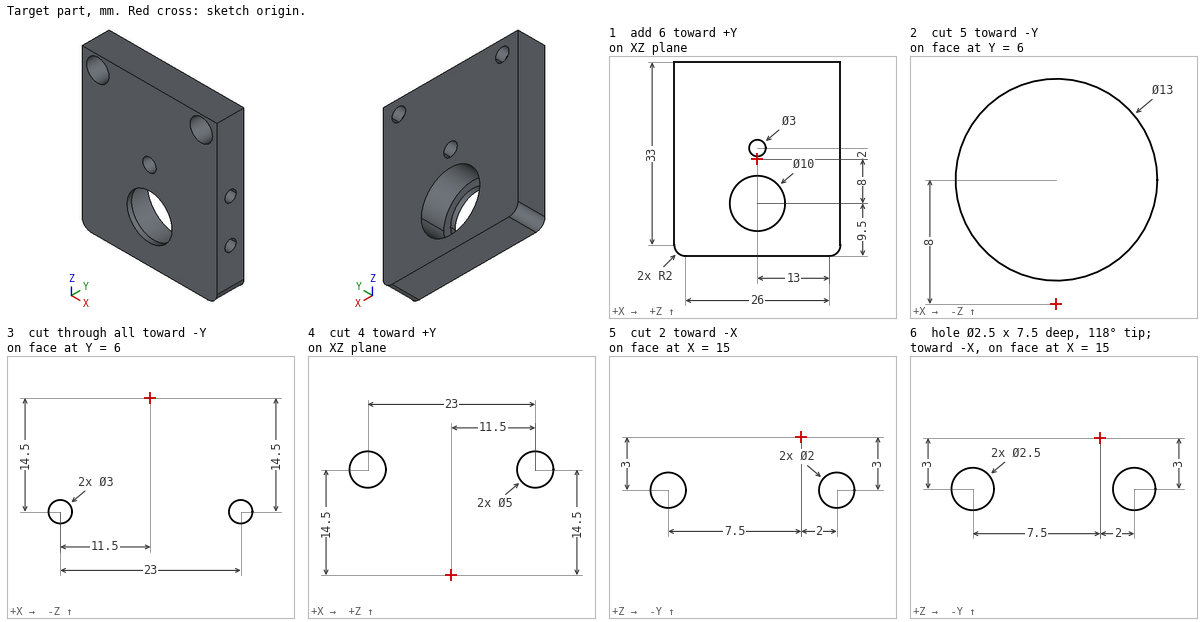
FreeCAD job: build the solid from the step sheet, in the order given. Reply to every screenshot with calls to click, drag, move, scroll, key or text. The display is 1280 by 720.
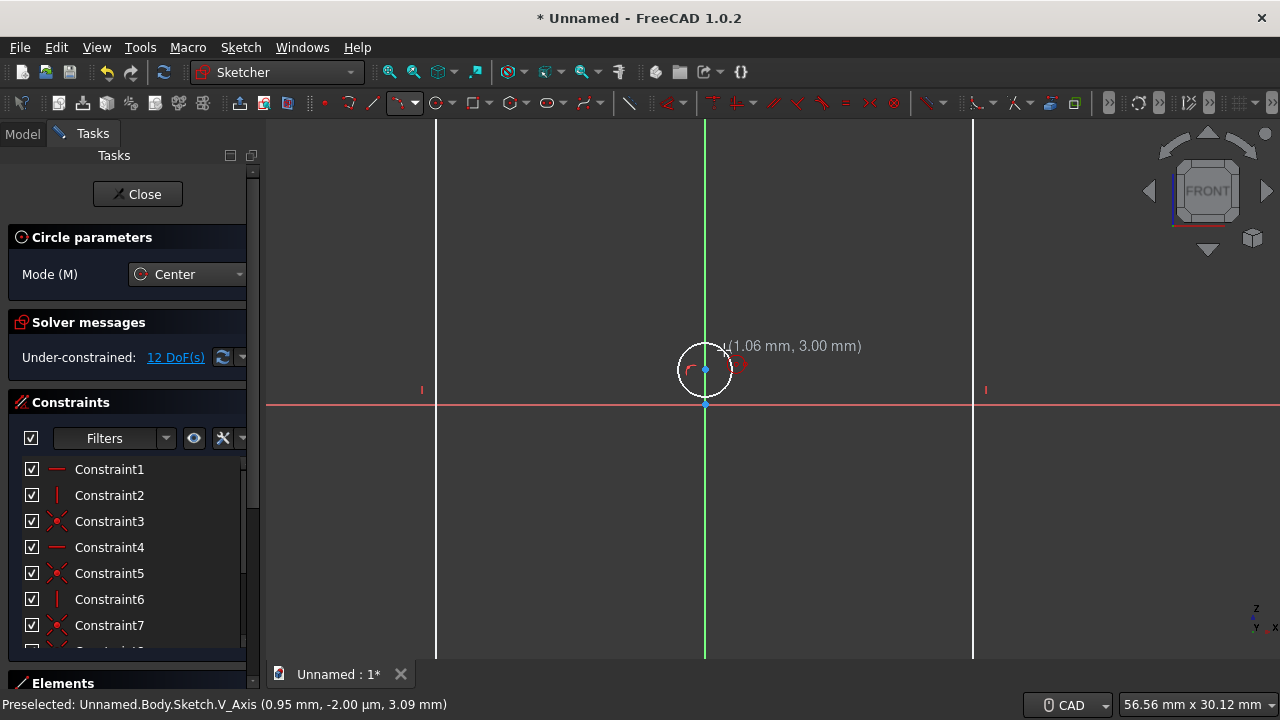
click(705, 548)
click(768, 485)
key(Escape)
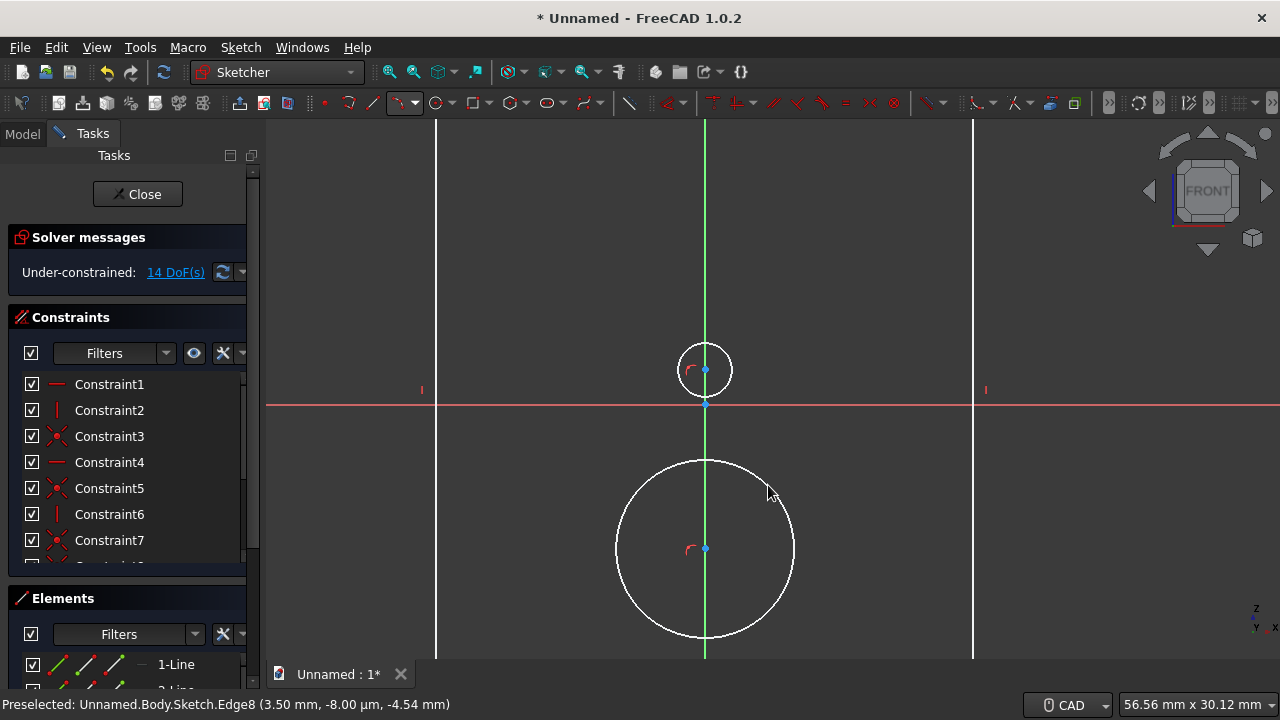
scroll(704, 370, down, 3)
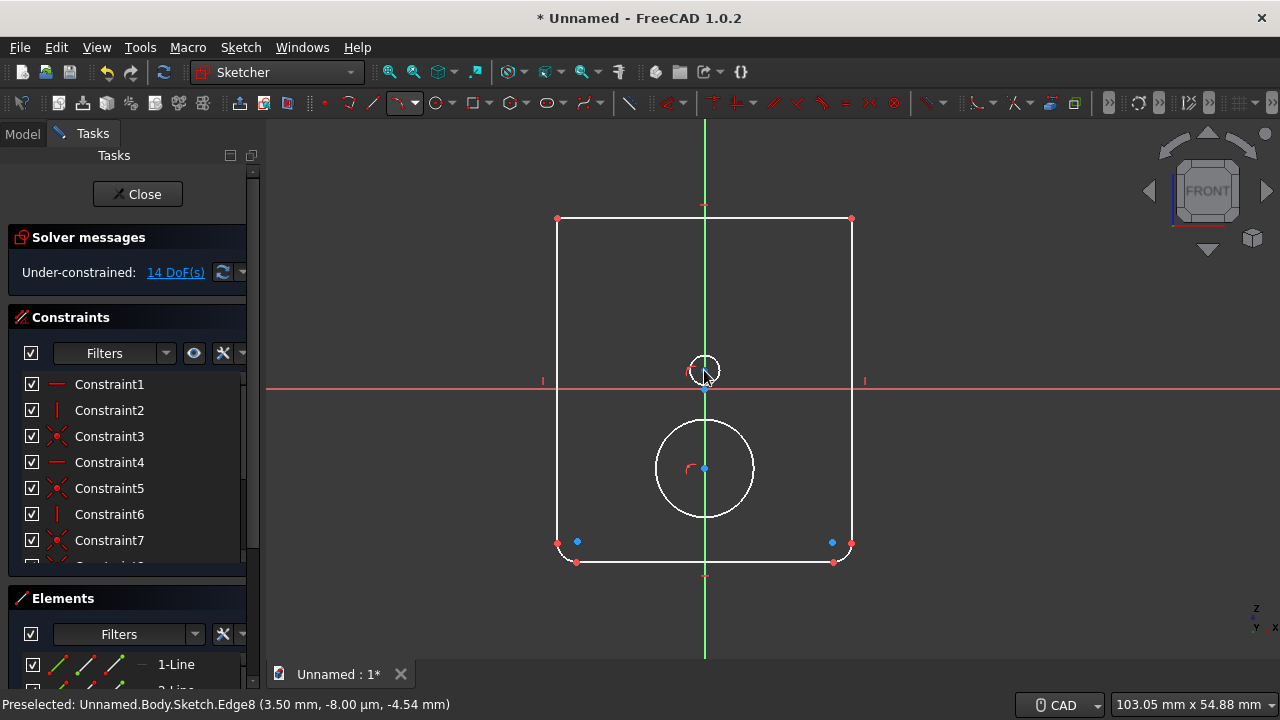
click(756, 562)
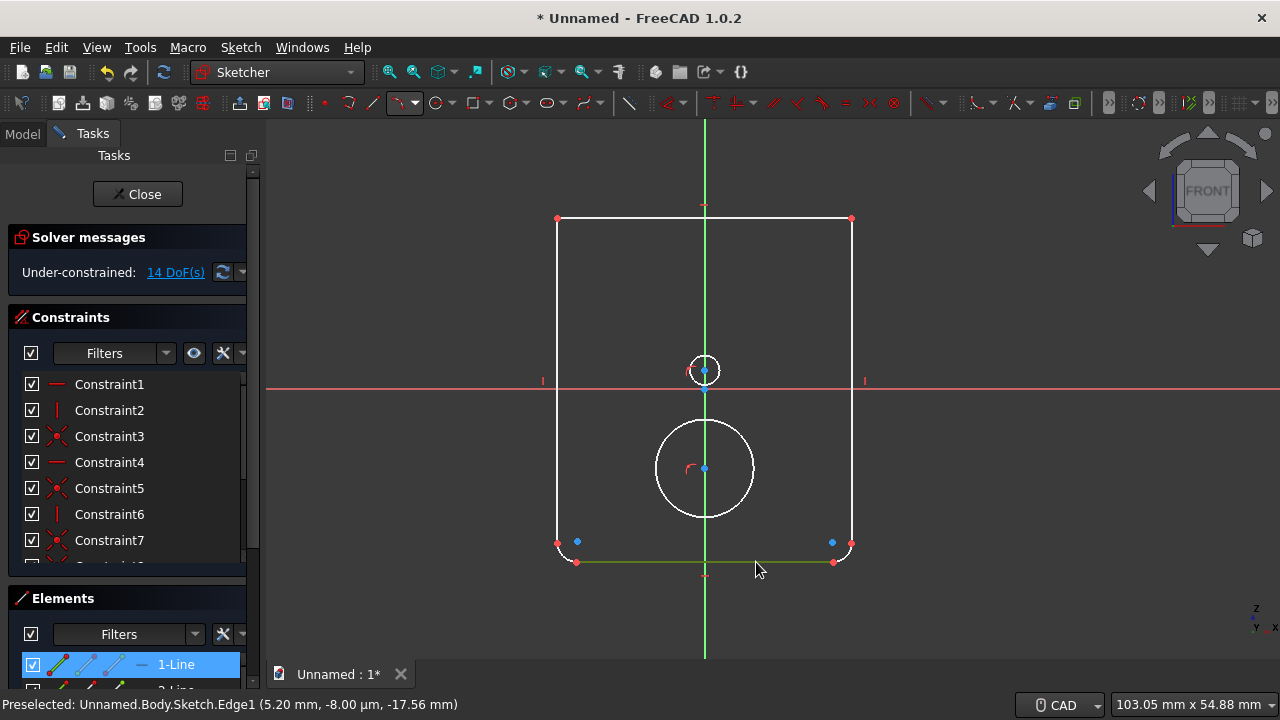
click(563, 556)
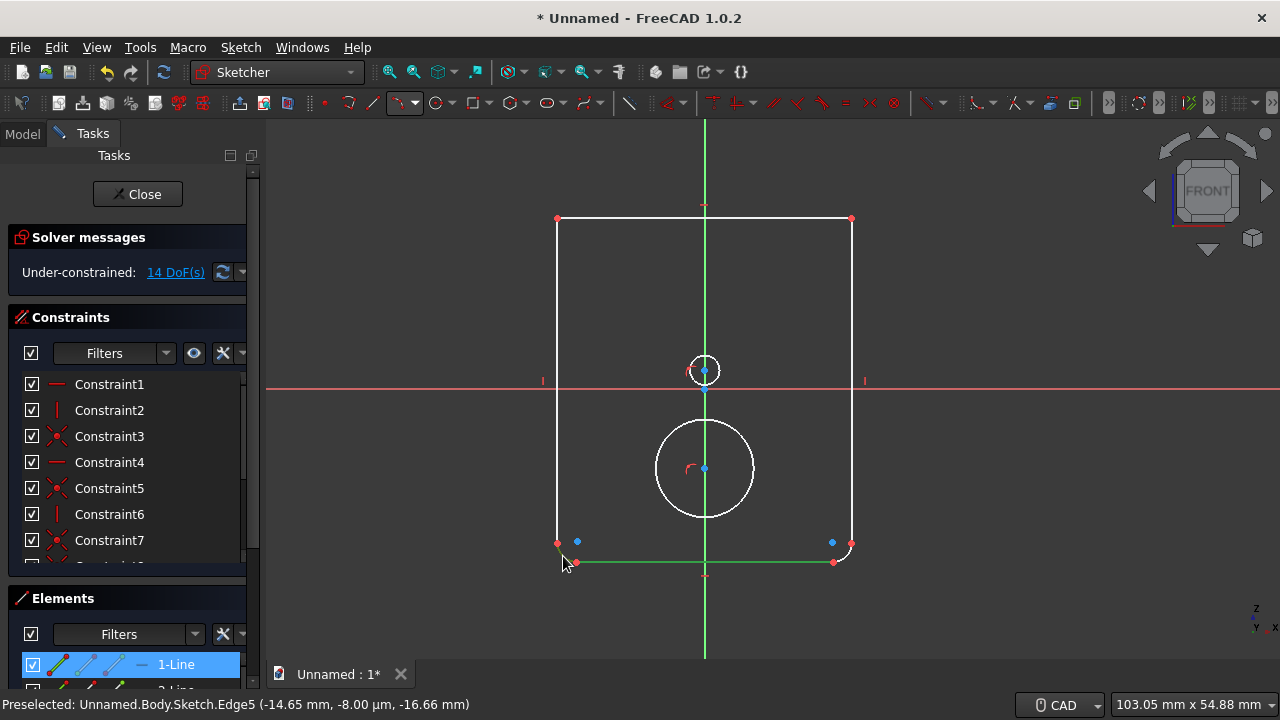
key(t)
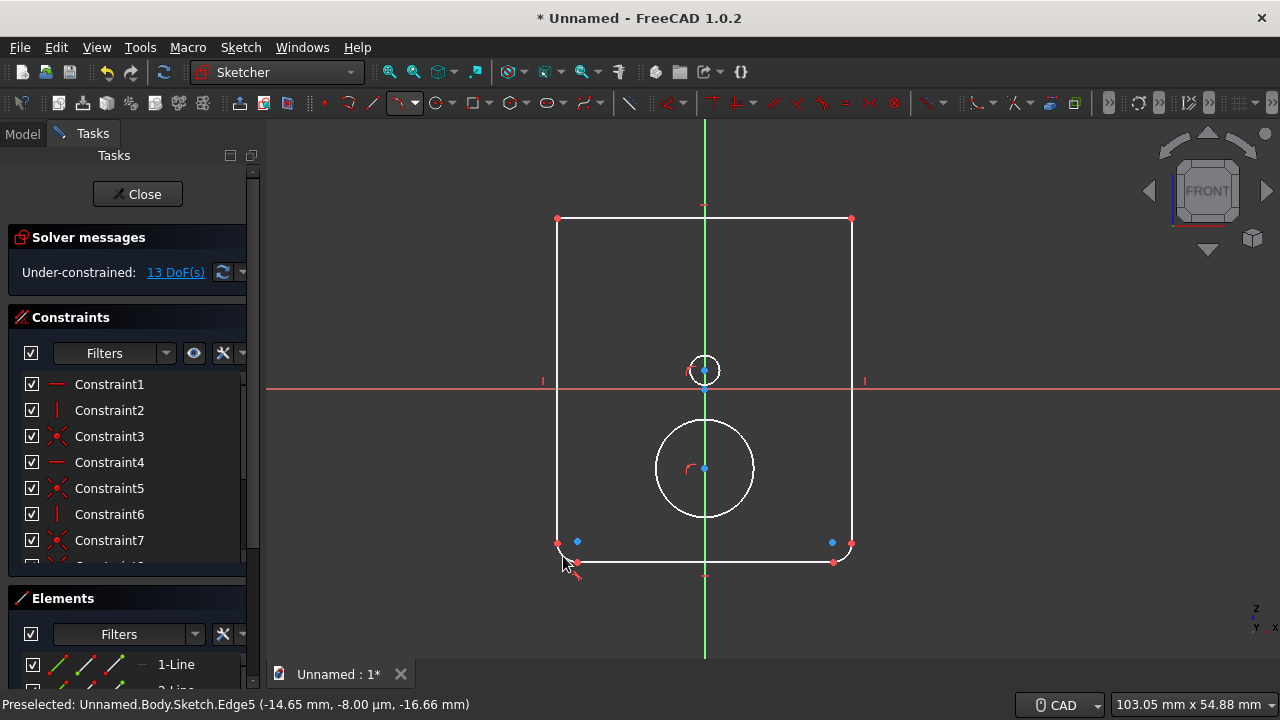
click(756, 562)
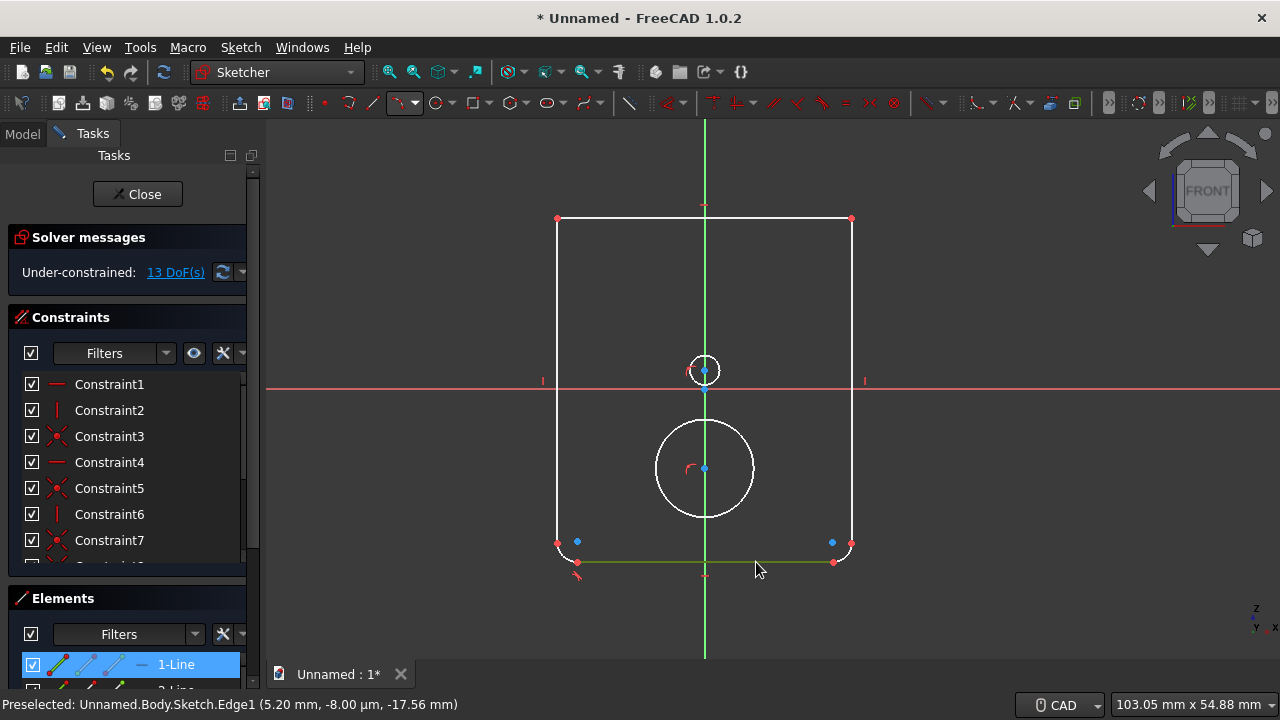
click(846, 556)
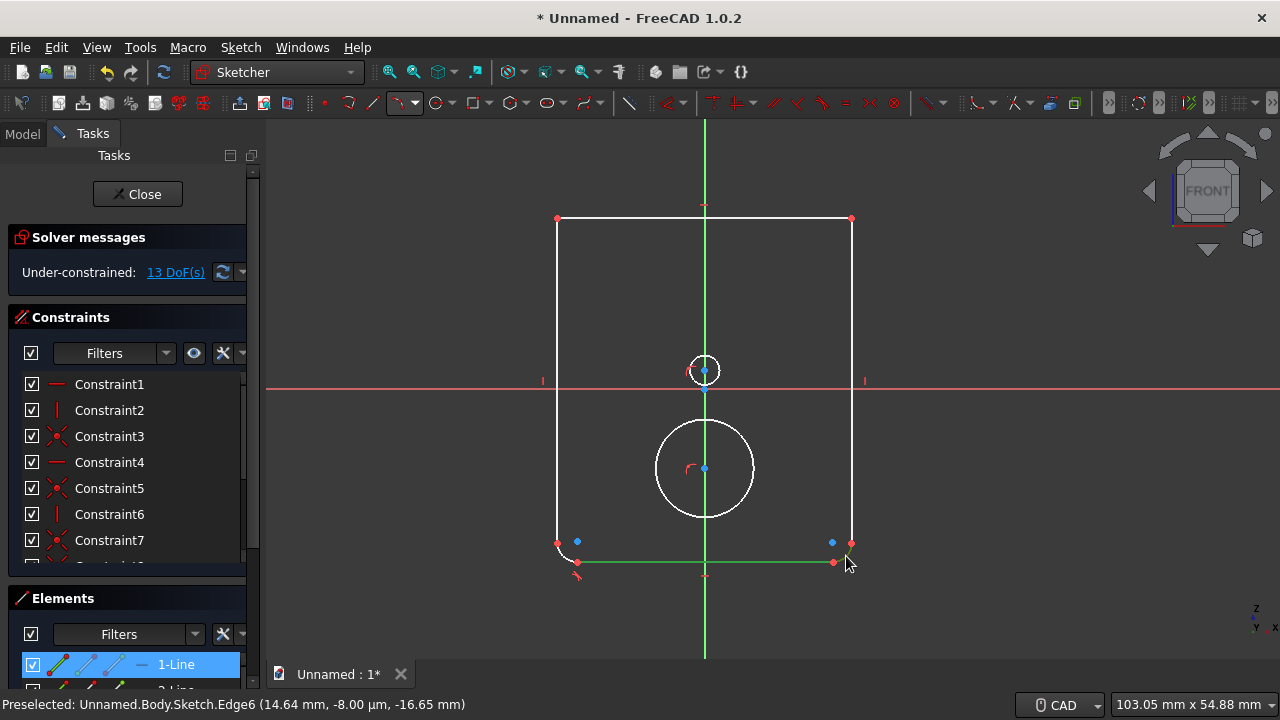
key(t)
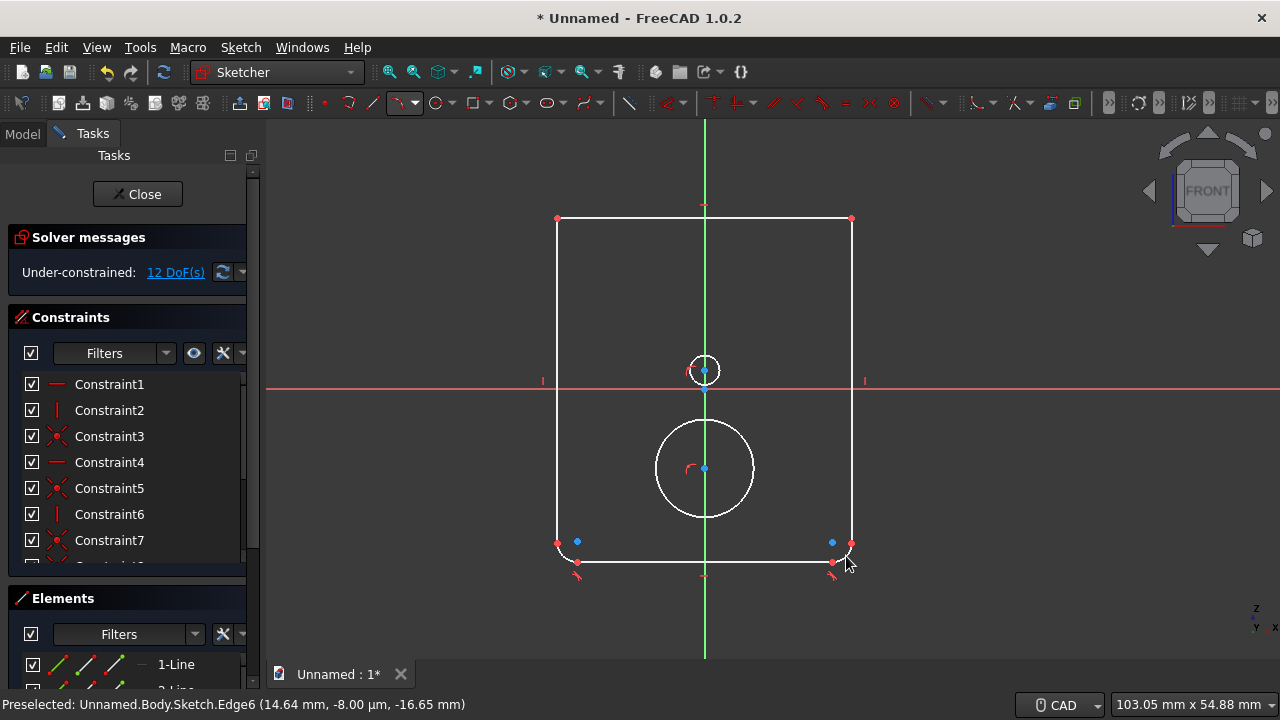
click(557, 446)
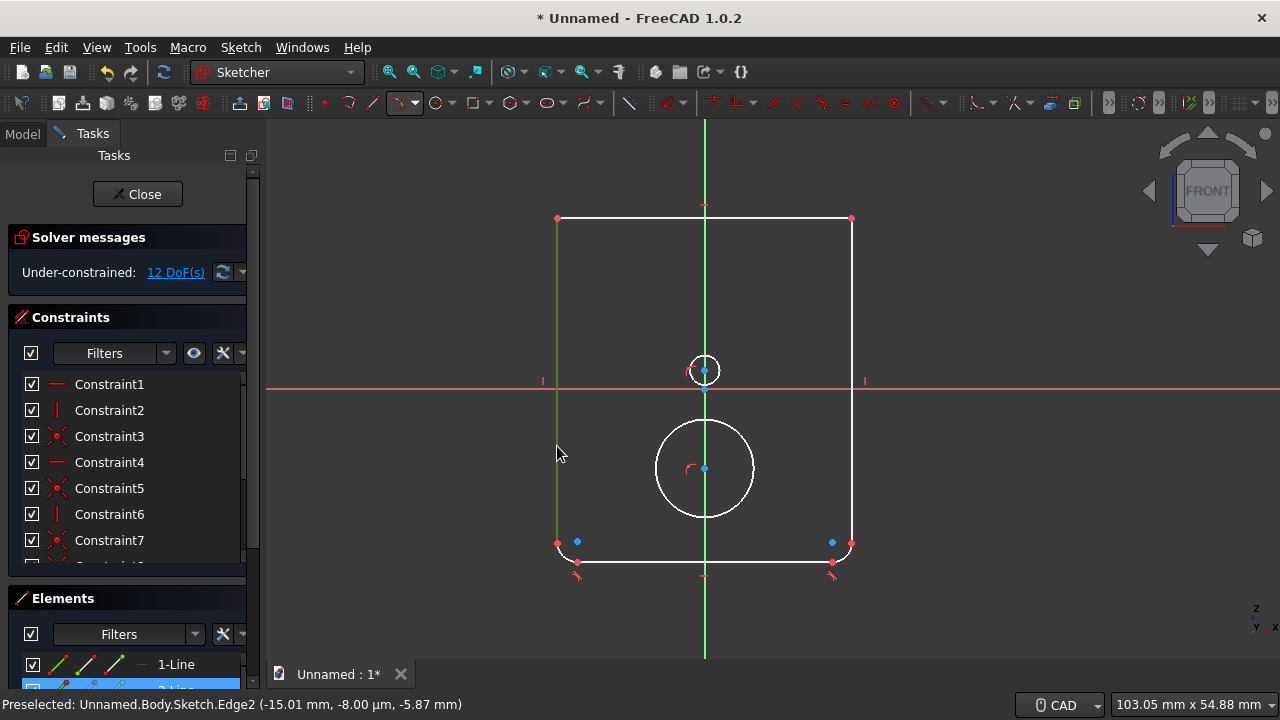
scroll(560, 552, up, 3)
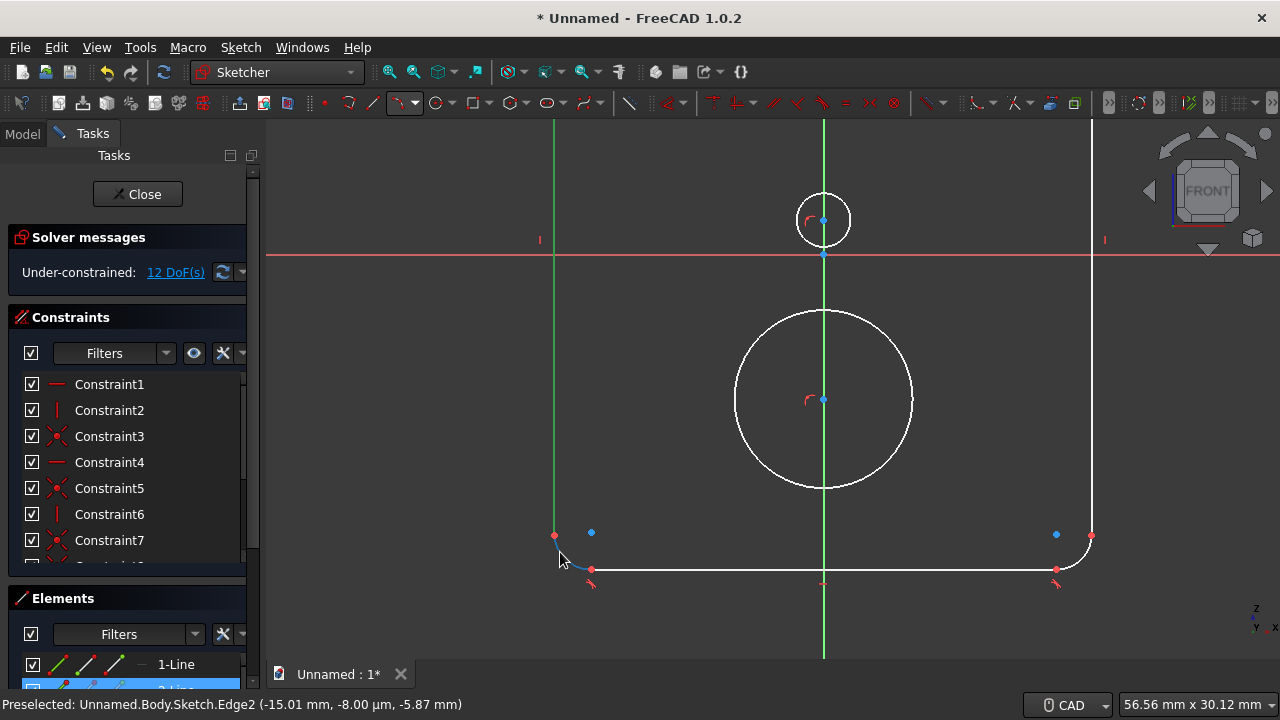
click(559, 551)